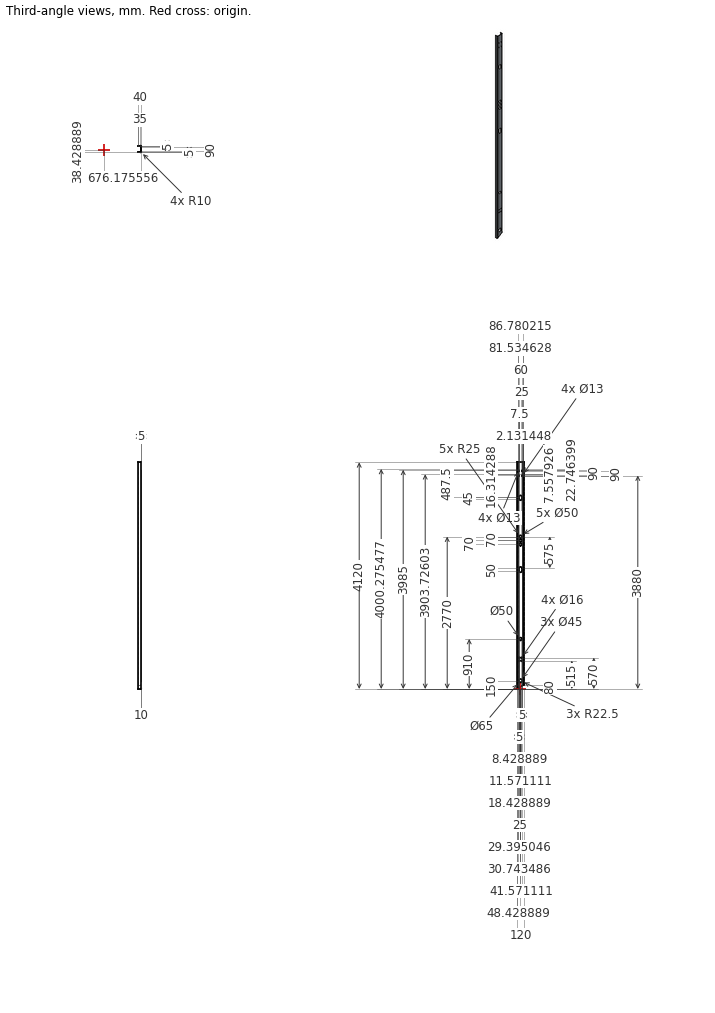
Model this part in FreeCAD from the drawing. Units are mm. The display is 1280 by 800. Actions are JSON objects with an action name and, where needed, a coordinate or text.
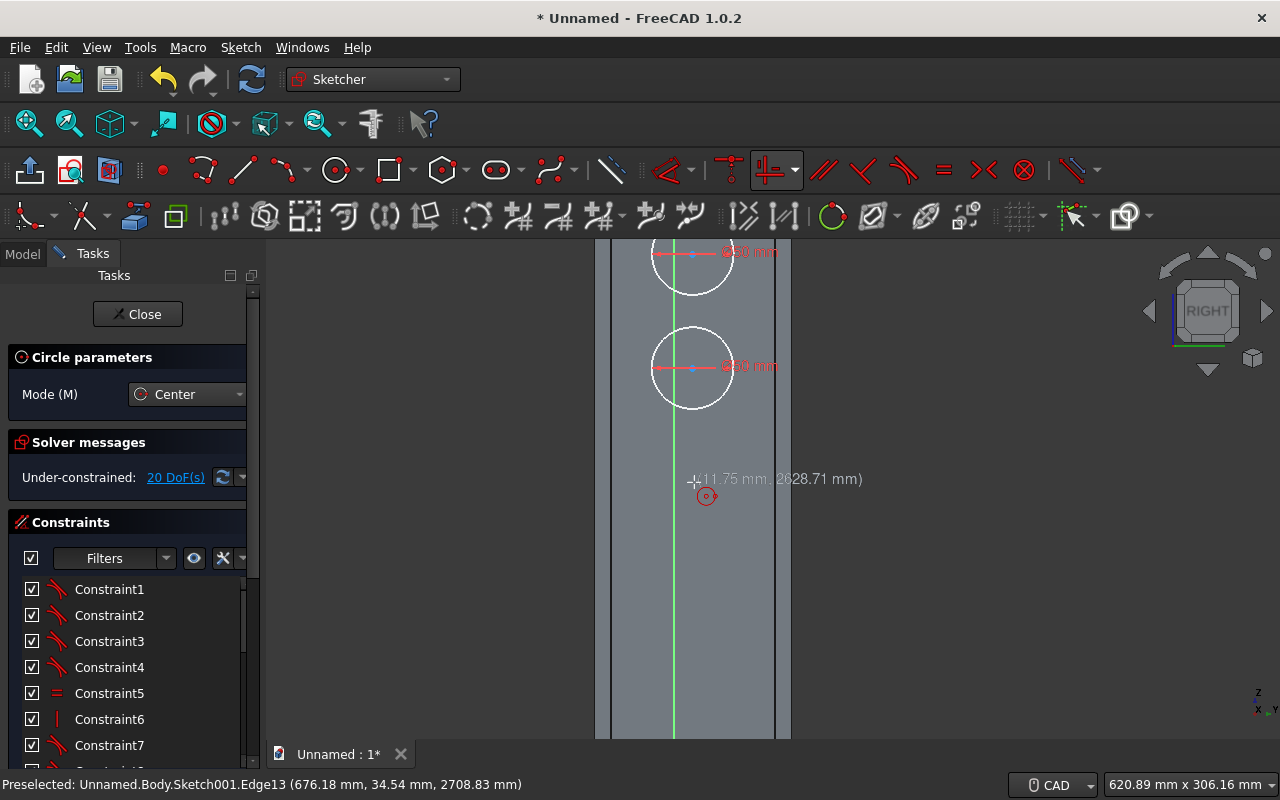
{"action": "left_click", "coordinate": [693, 482]}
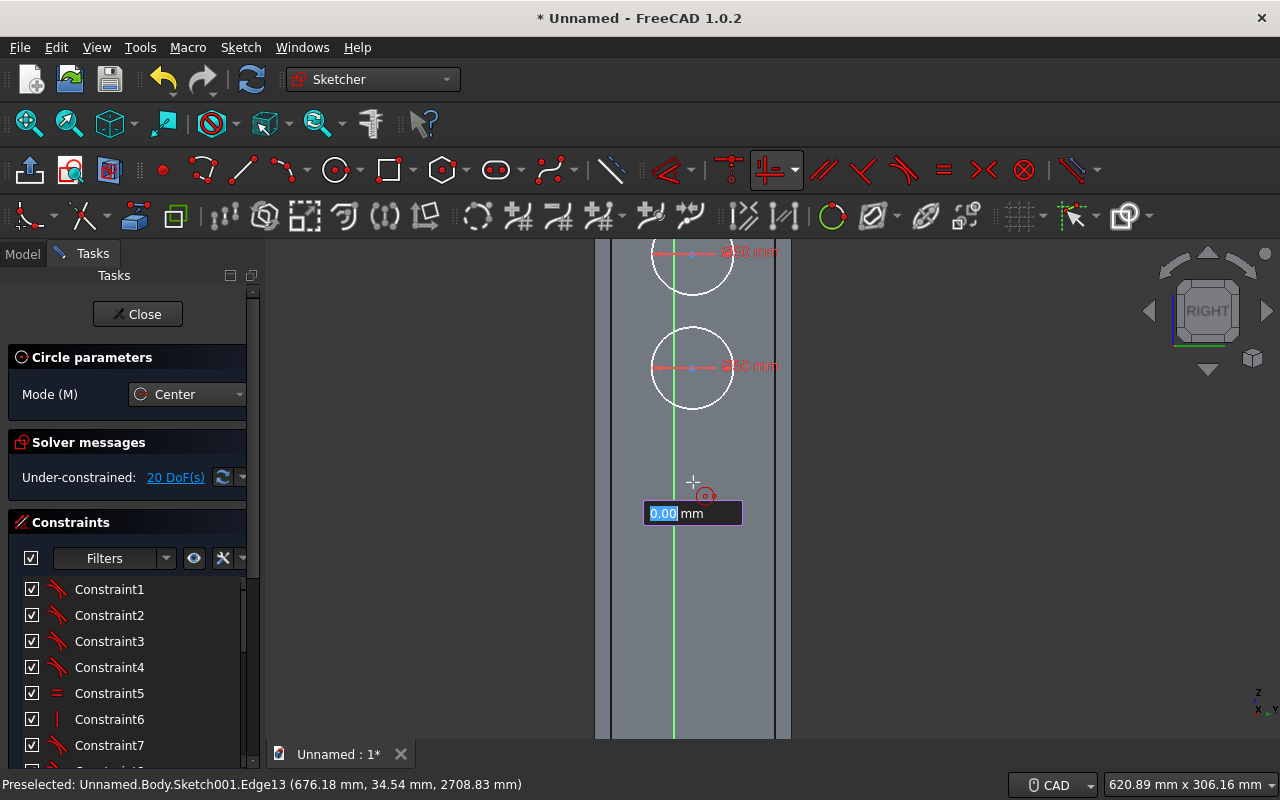
{"action": "scroll", "coordinate": [705, 435], "scroll_direction": "down", "scroll_amount": 15}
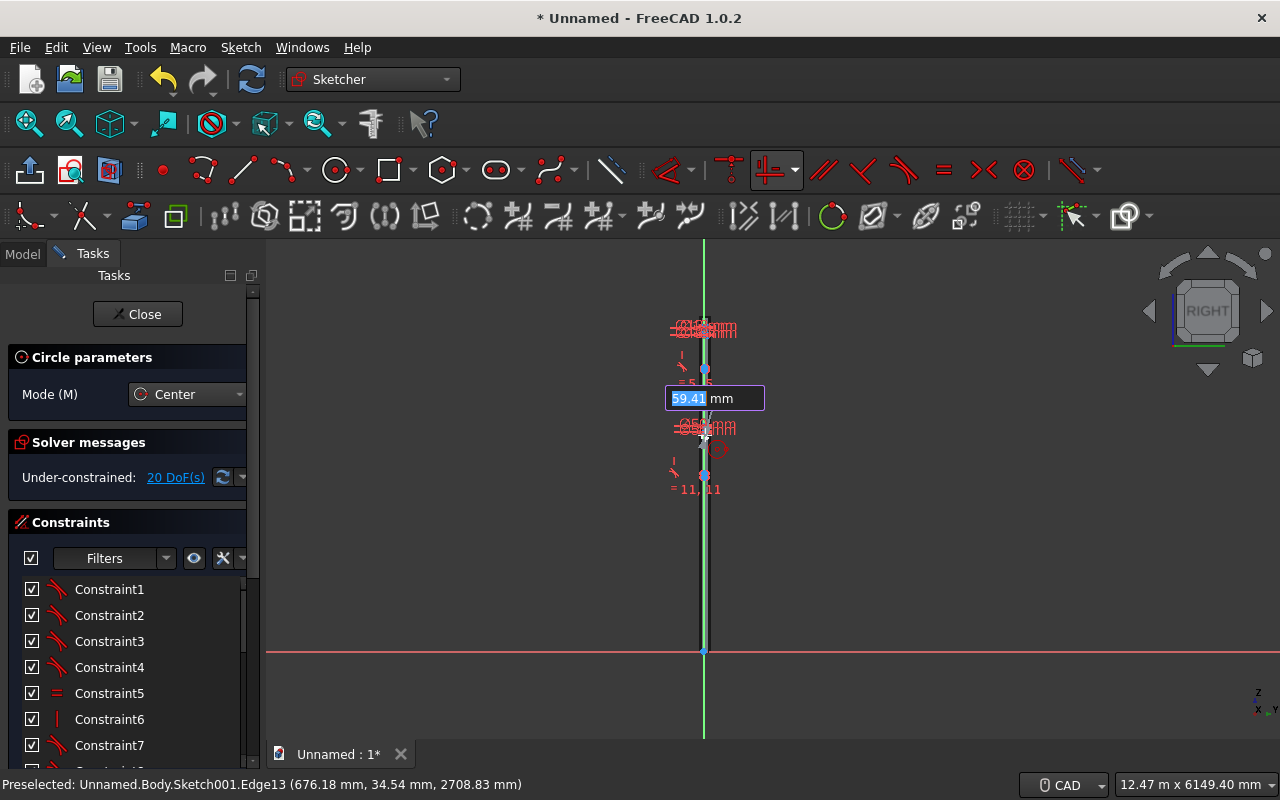
{"action": "scroll", "coordinate": [706, 436], "scroll_direction": "up", "scroll_amount": 10}
{"action": "mouse_move", "coordinate": [705, 435]}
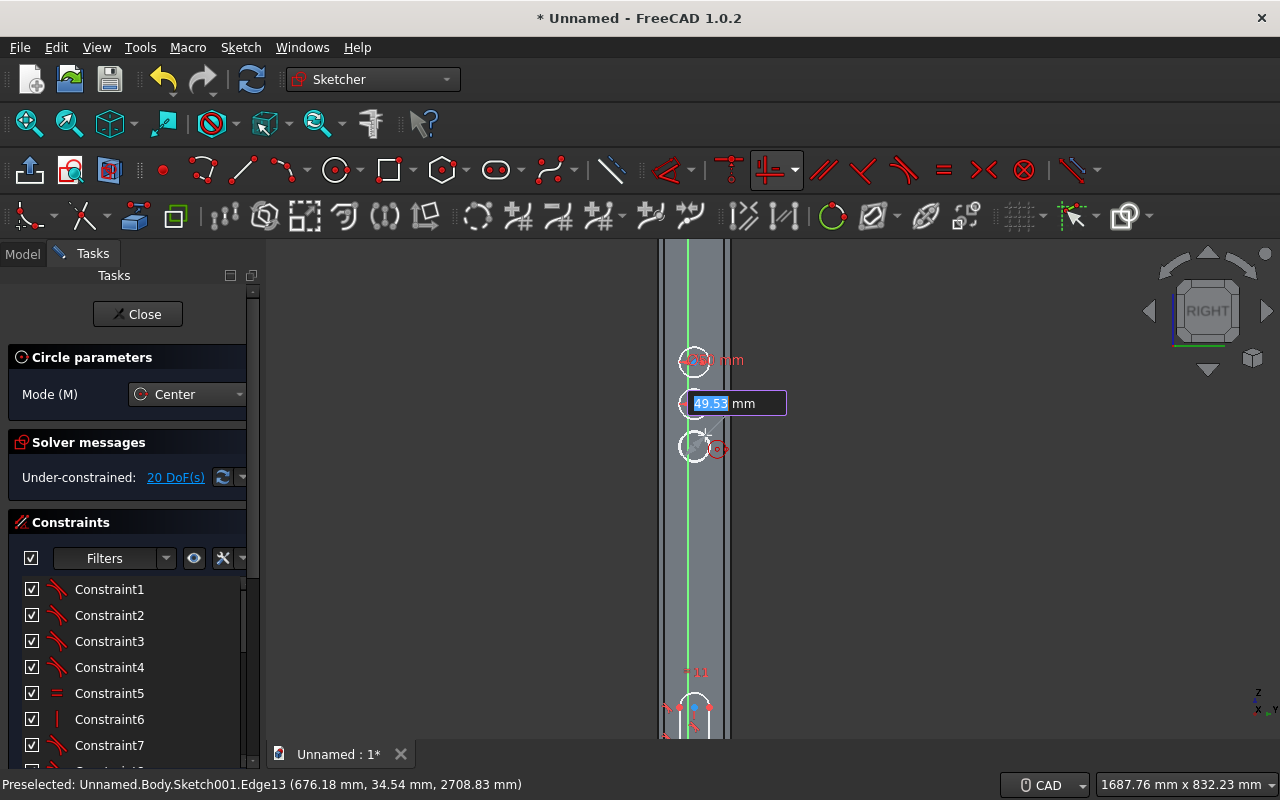
{"action": "type", "text": "50"}
{"action": "key", "text": "Return"}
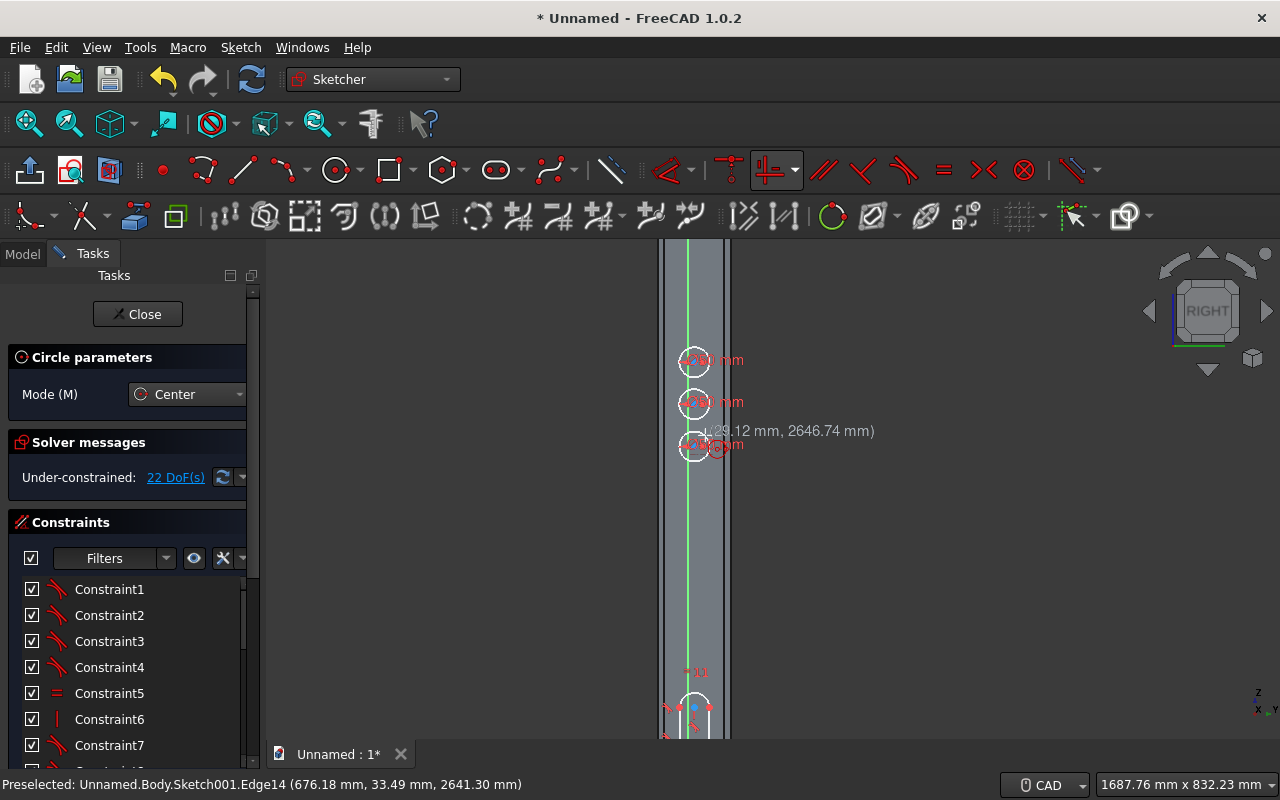
{"action": "scroll", "coordinate": [706, 436], "scroll_direction": "down", "scroll_amount": 10}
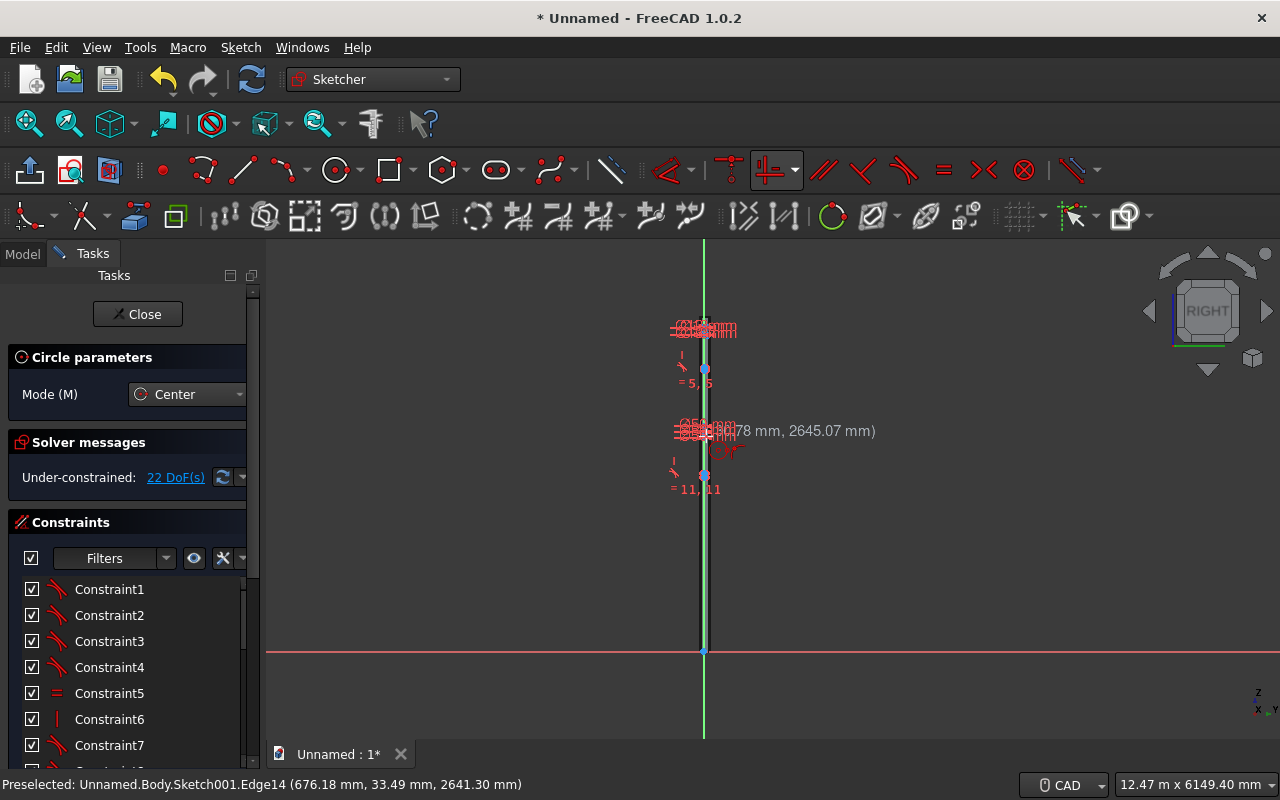
{"action": "scroll", "coordinate": [705, 639], "scroll_direction": "up", "scroll_amount": 15}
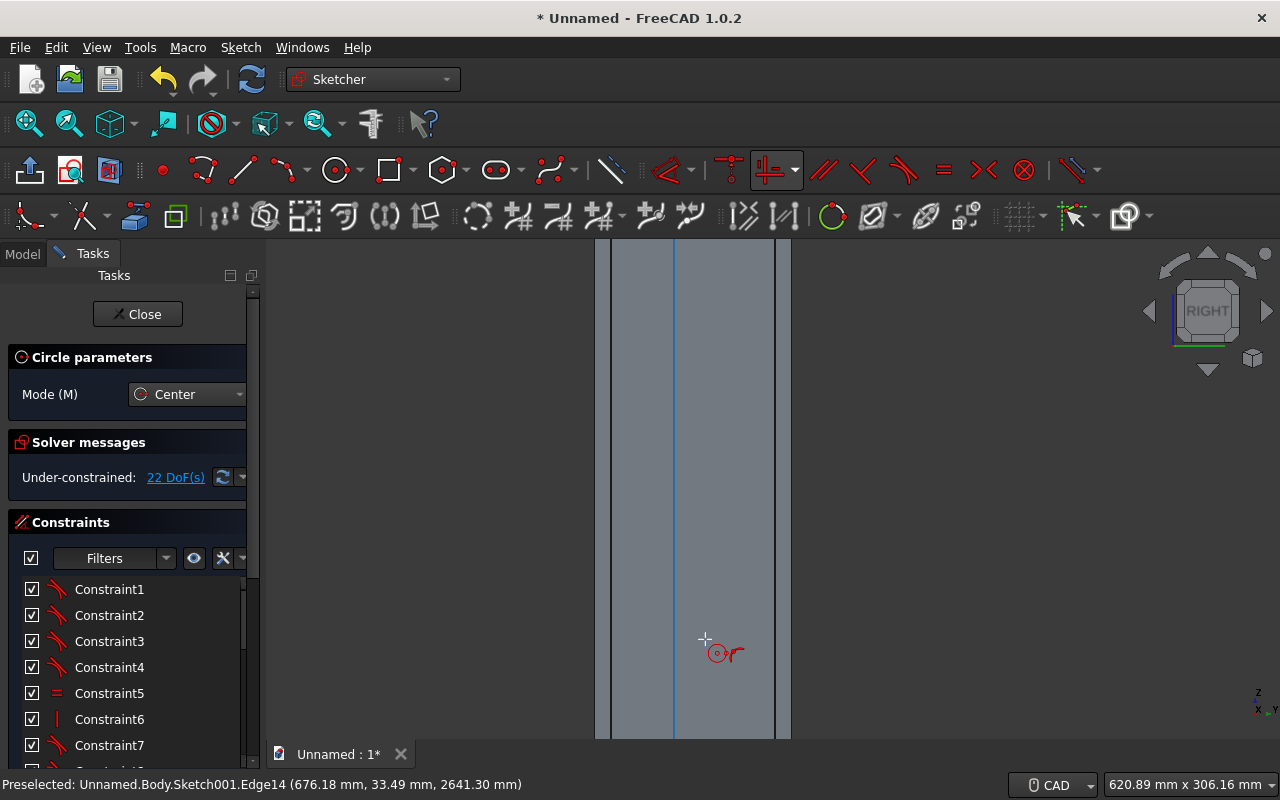
{"action": "left_click", "coordinate": [693, 631]}
{"action": "mouse_move", "coordinate": [719, 605]}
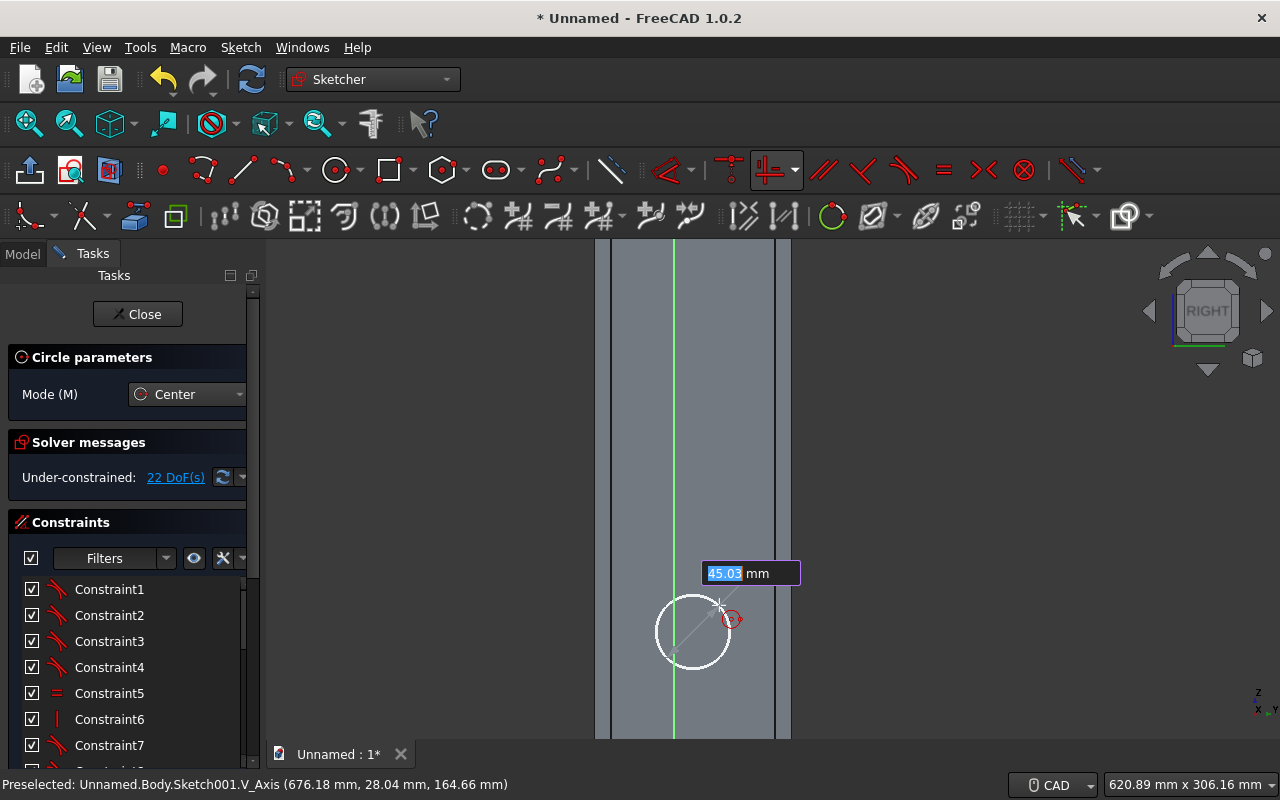
{"action": "type", "text": "45"}
{"action": "key", "text": "Return"}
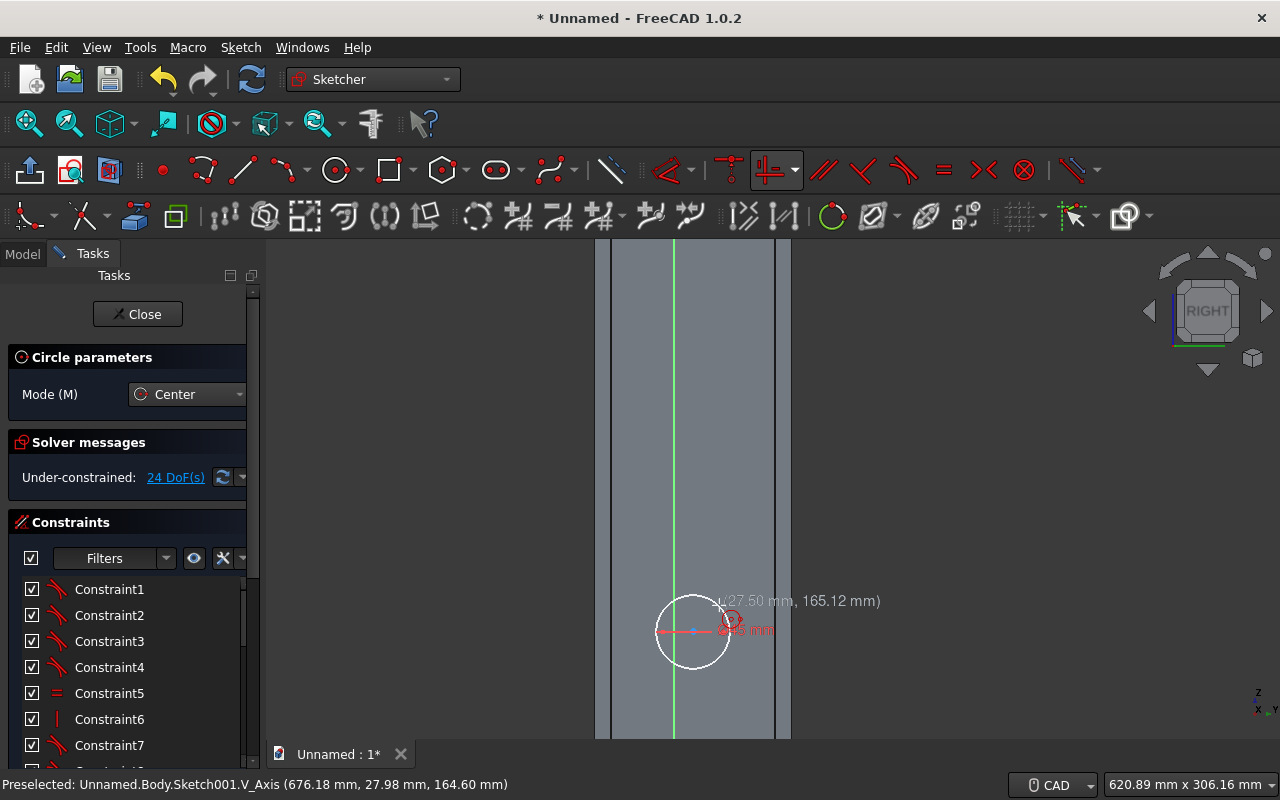
{"action": "scroll", "coordinate": [705, 640], "scroll_direction": "down", "scroll_amount": 15}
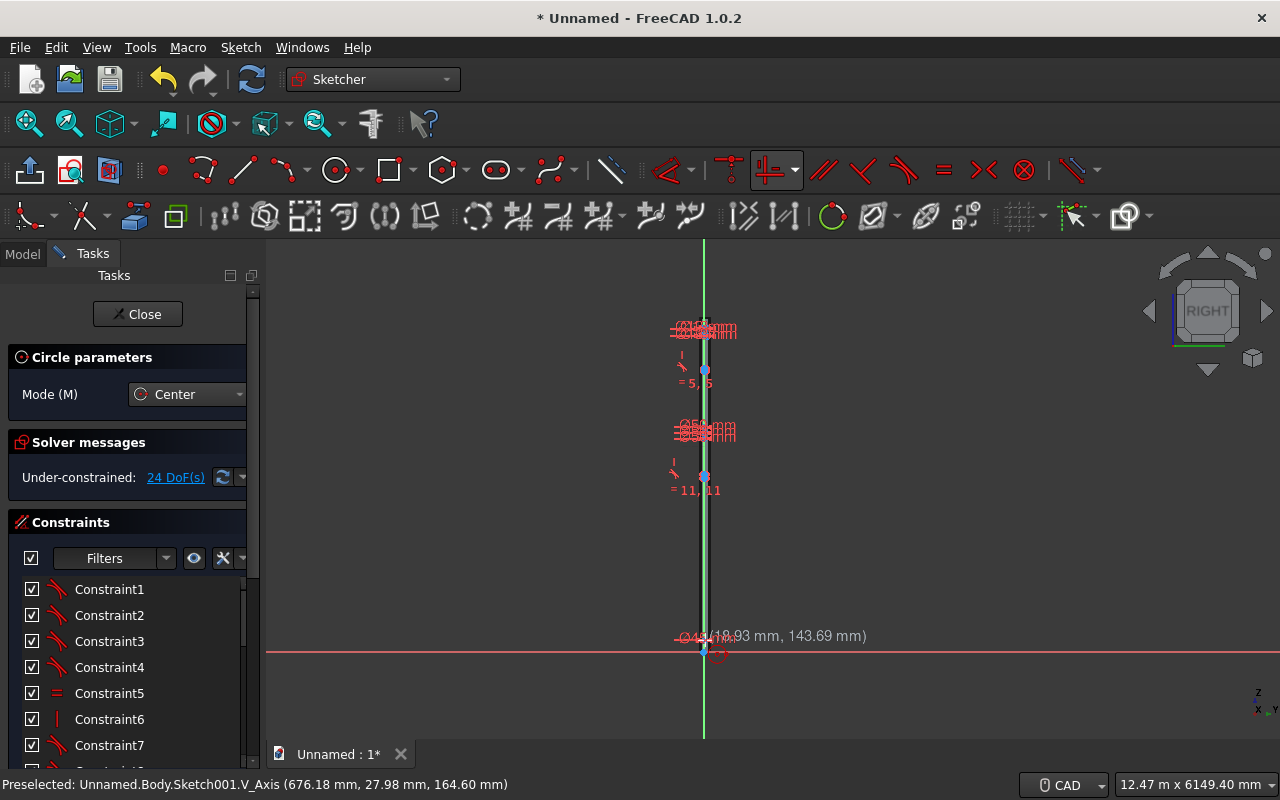
{"action": "scroll", "coordinate": [706, 606], "scroll_direction": "up", "scroll_amount": 18}